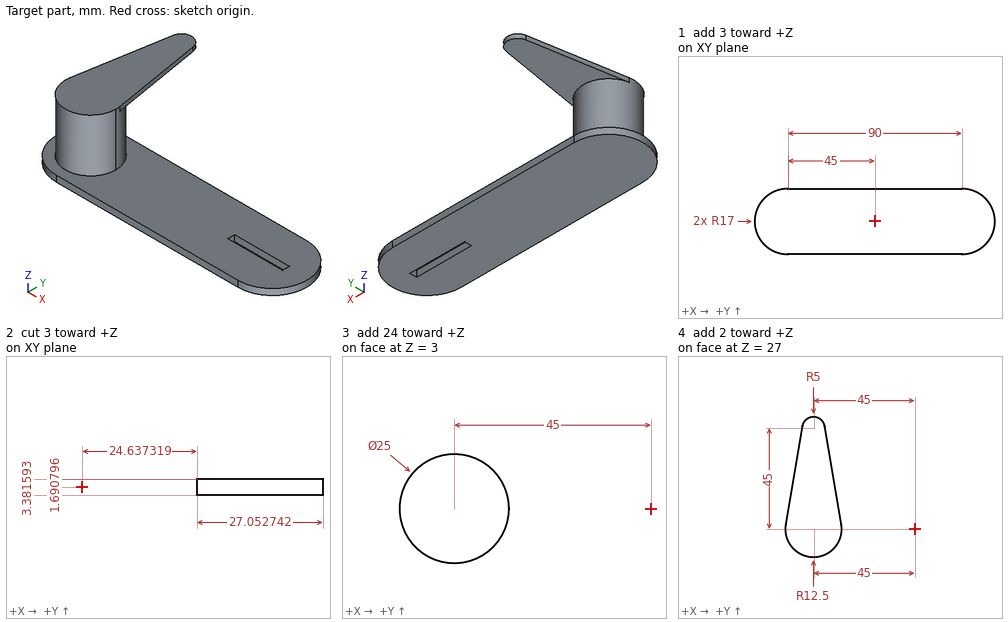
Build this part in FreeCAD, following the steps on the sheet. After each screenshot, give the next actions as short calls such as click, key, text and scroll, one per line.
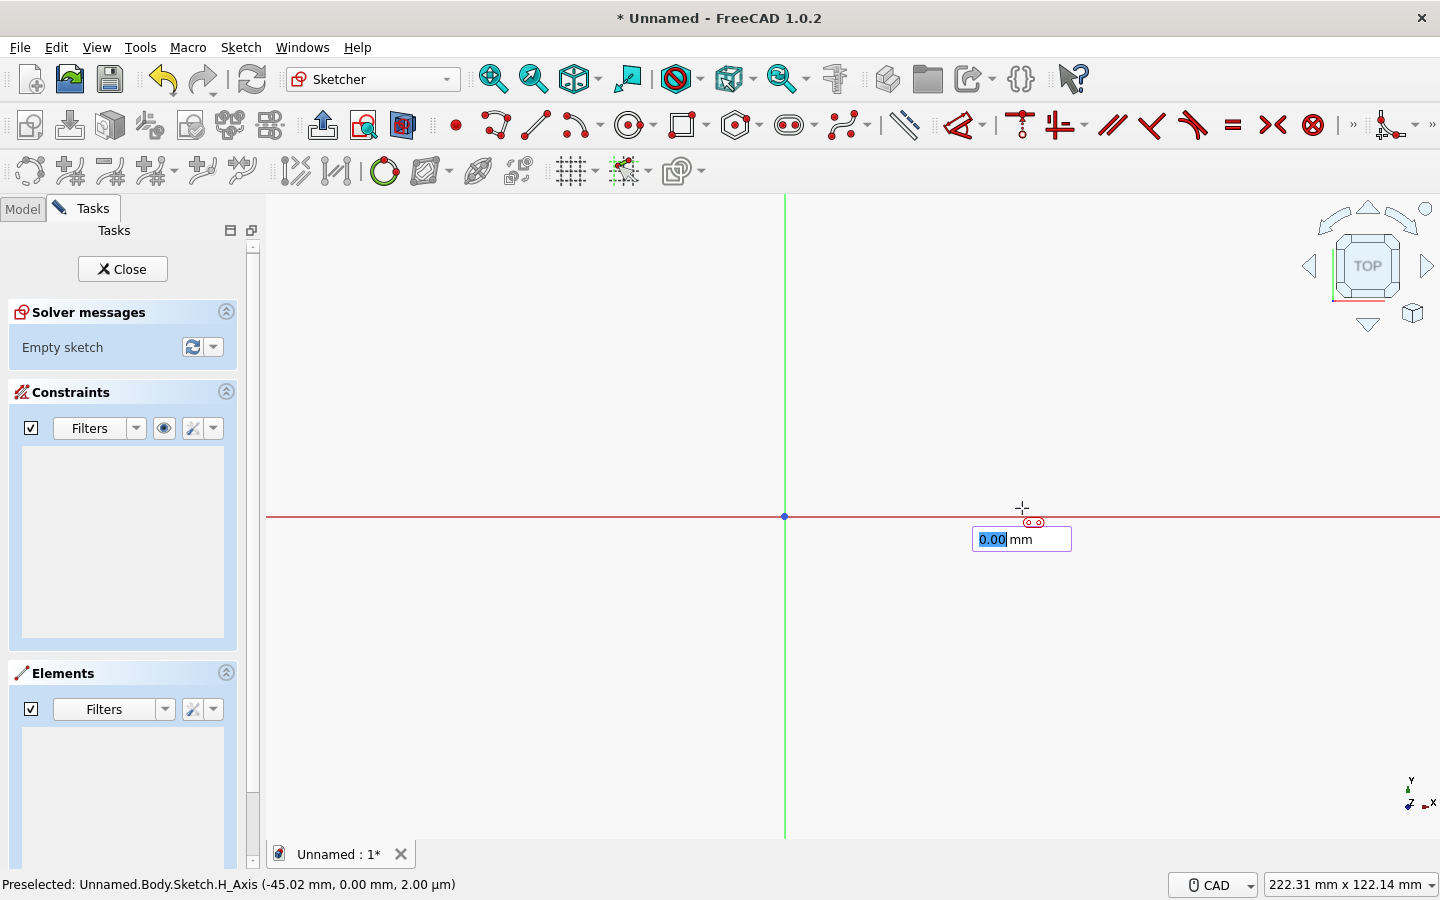
click(856, 427)
key(Escape)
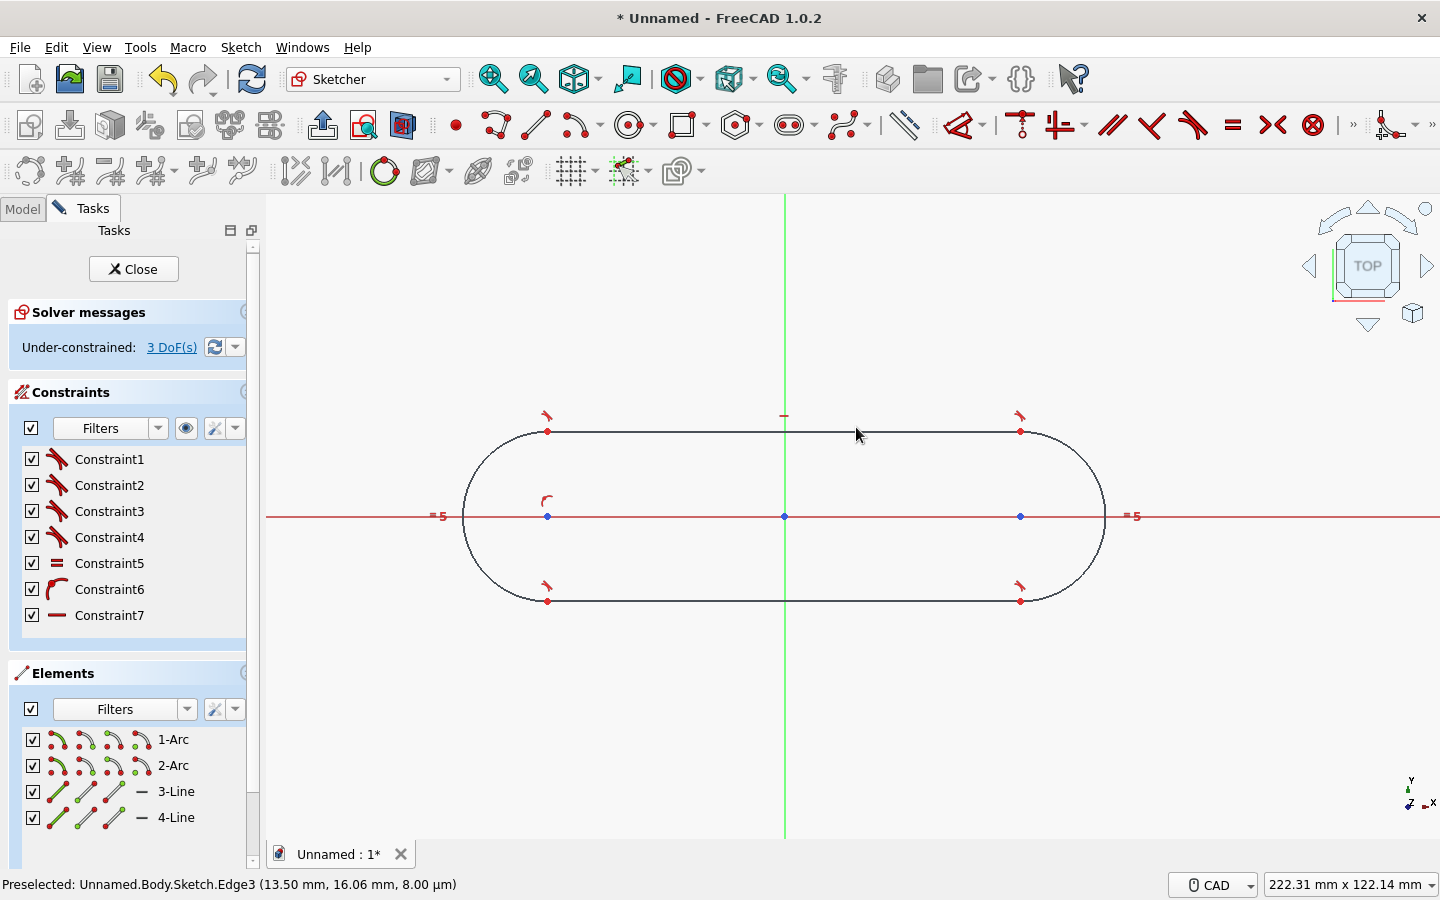
click(958, 126)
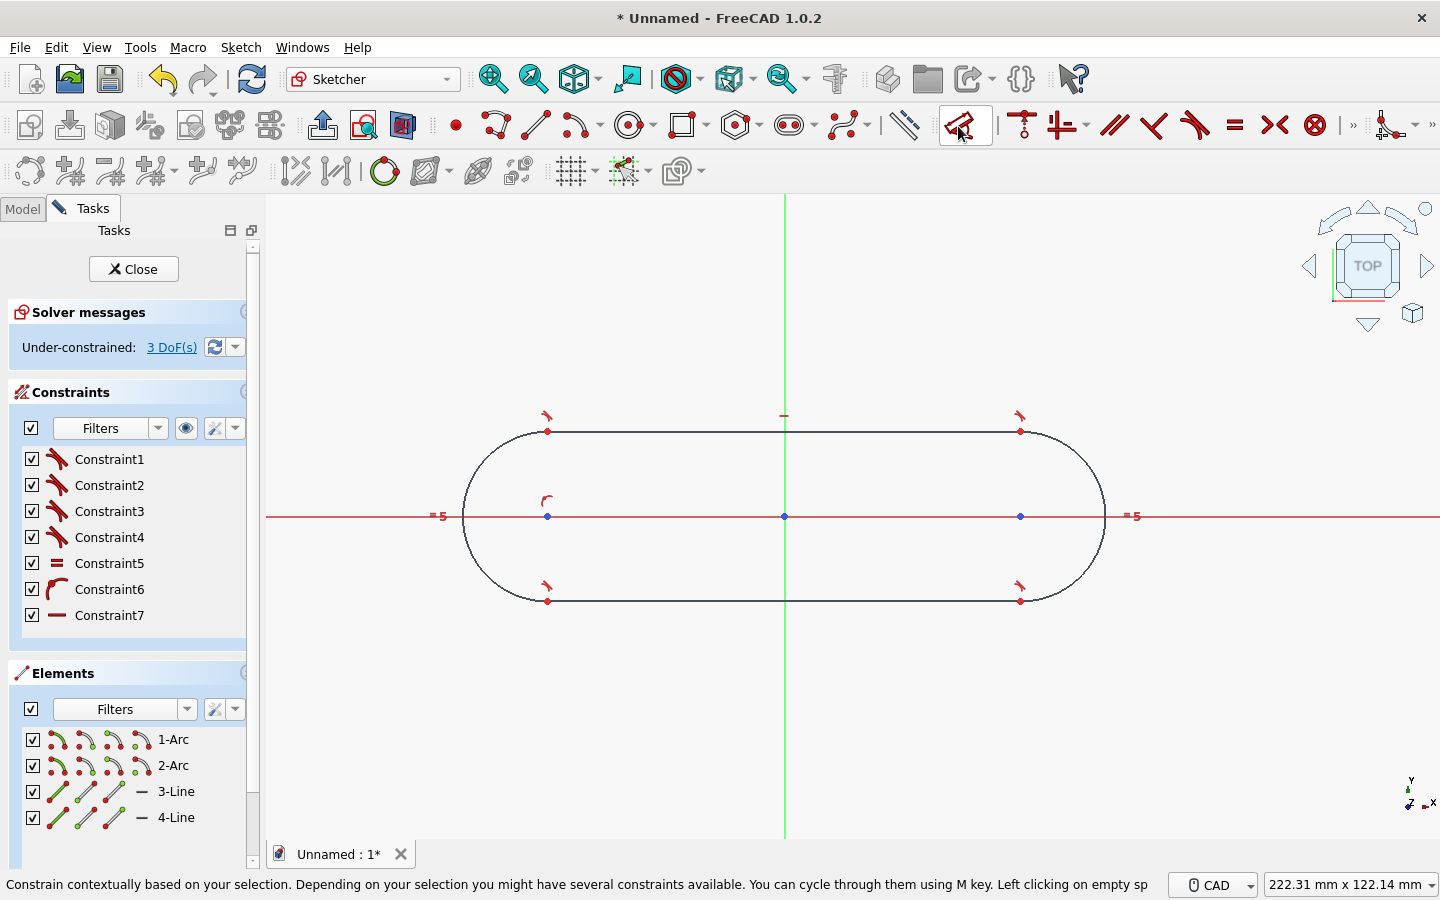
click(479, 467)
click(453, 448)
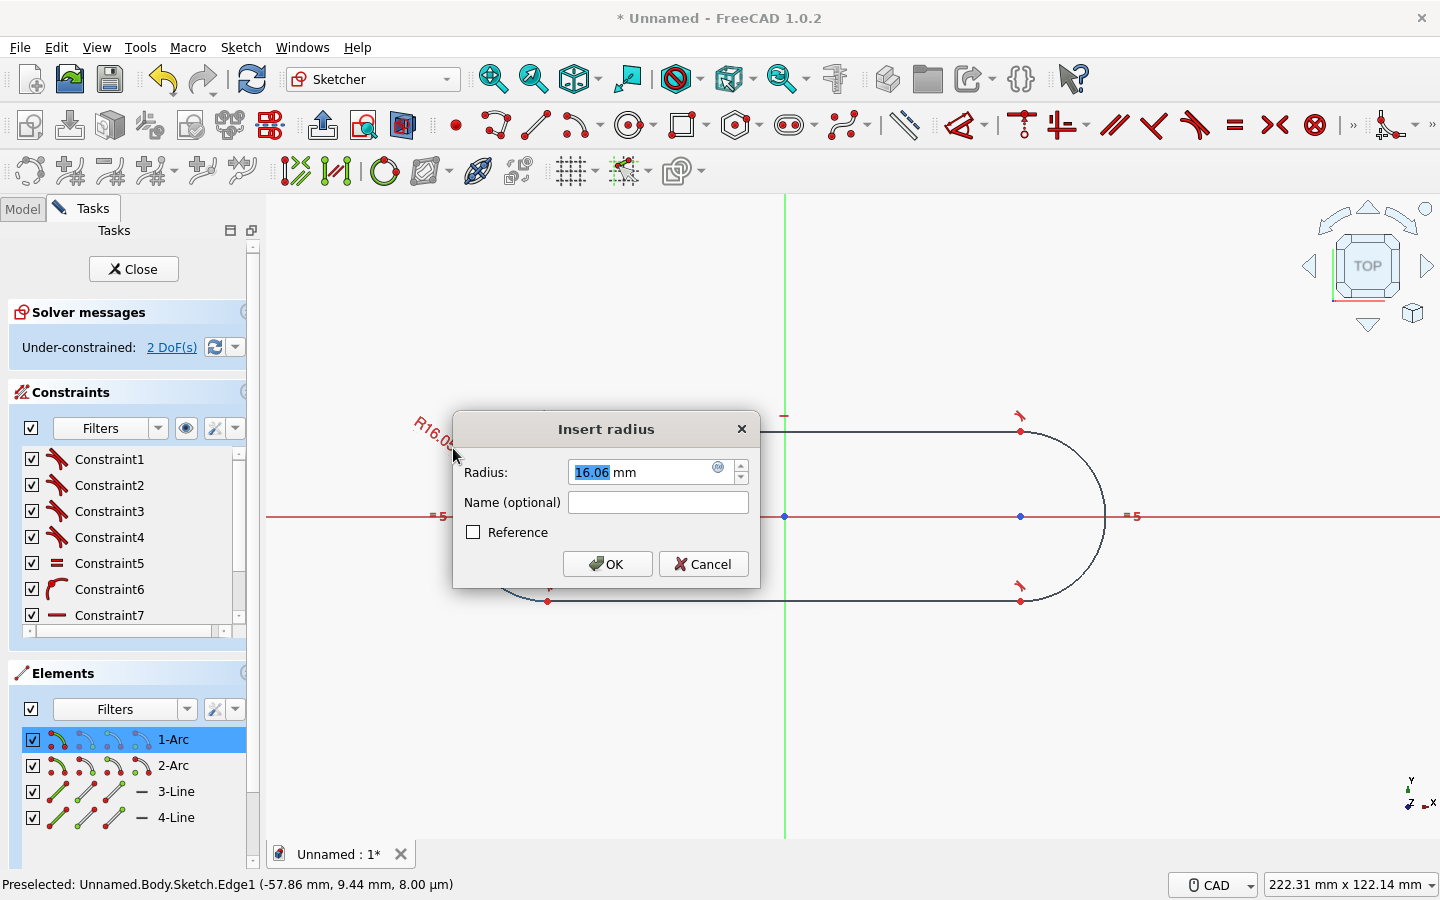
text(17)
key(Return)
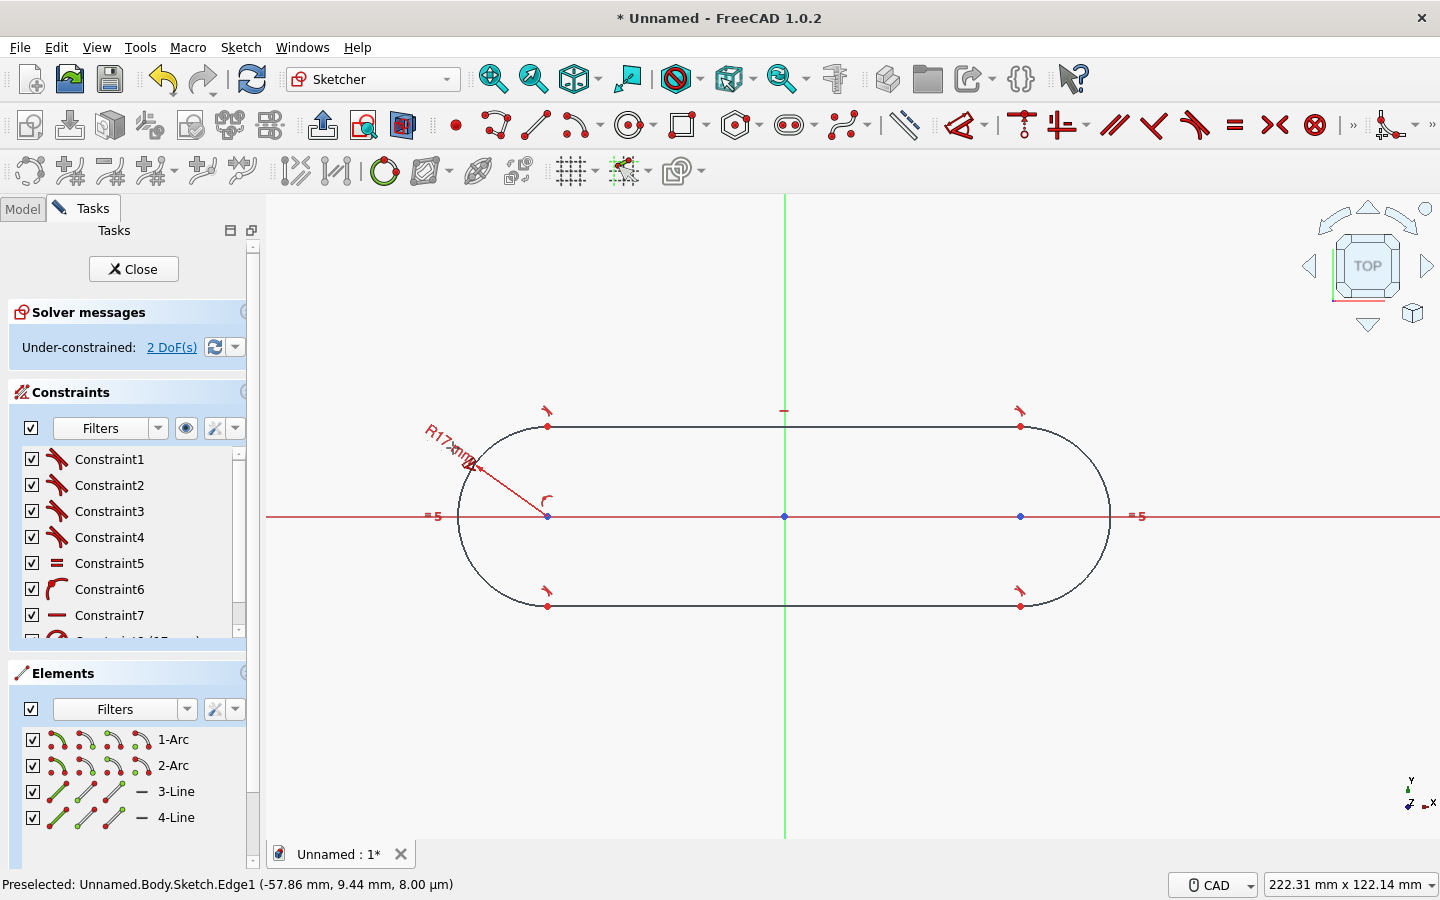
click(690, 427)
click(675, 393)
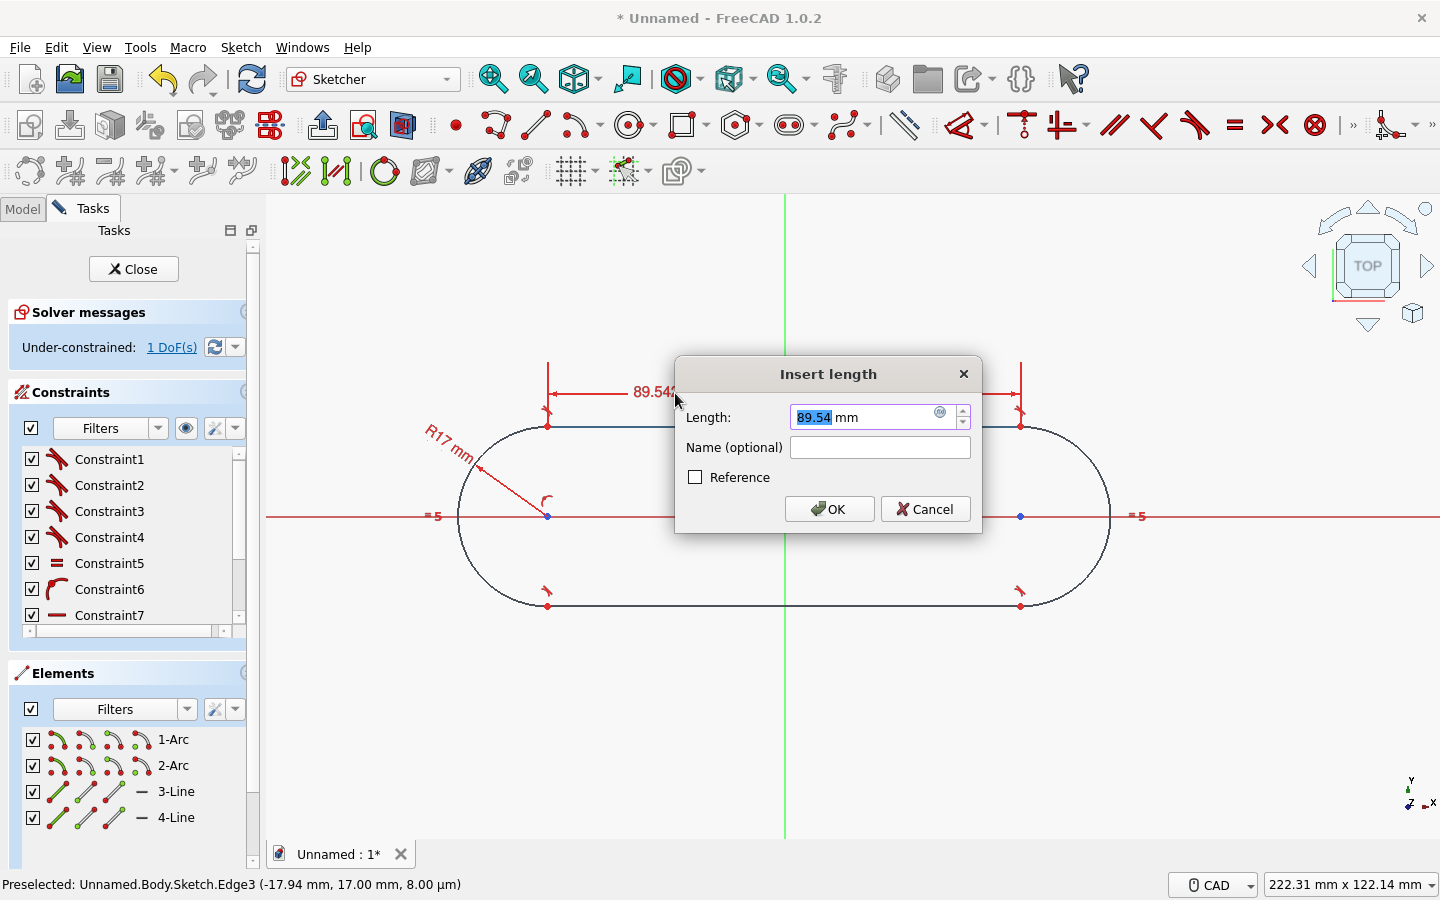
text(90)
key(Return)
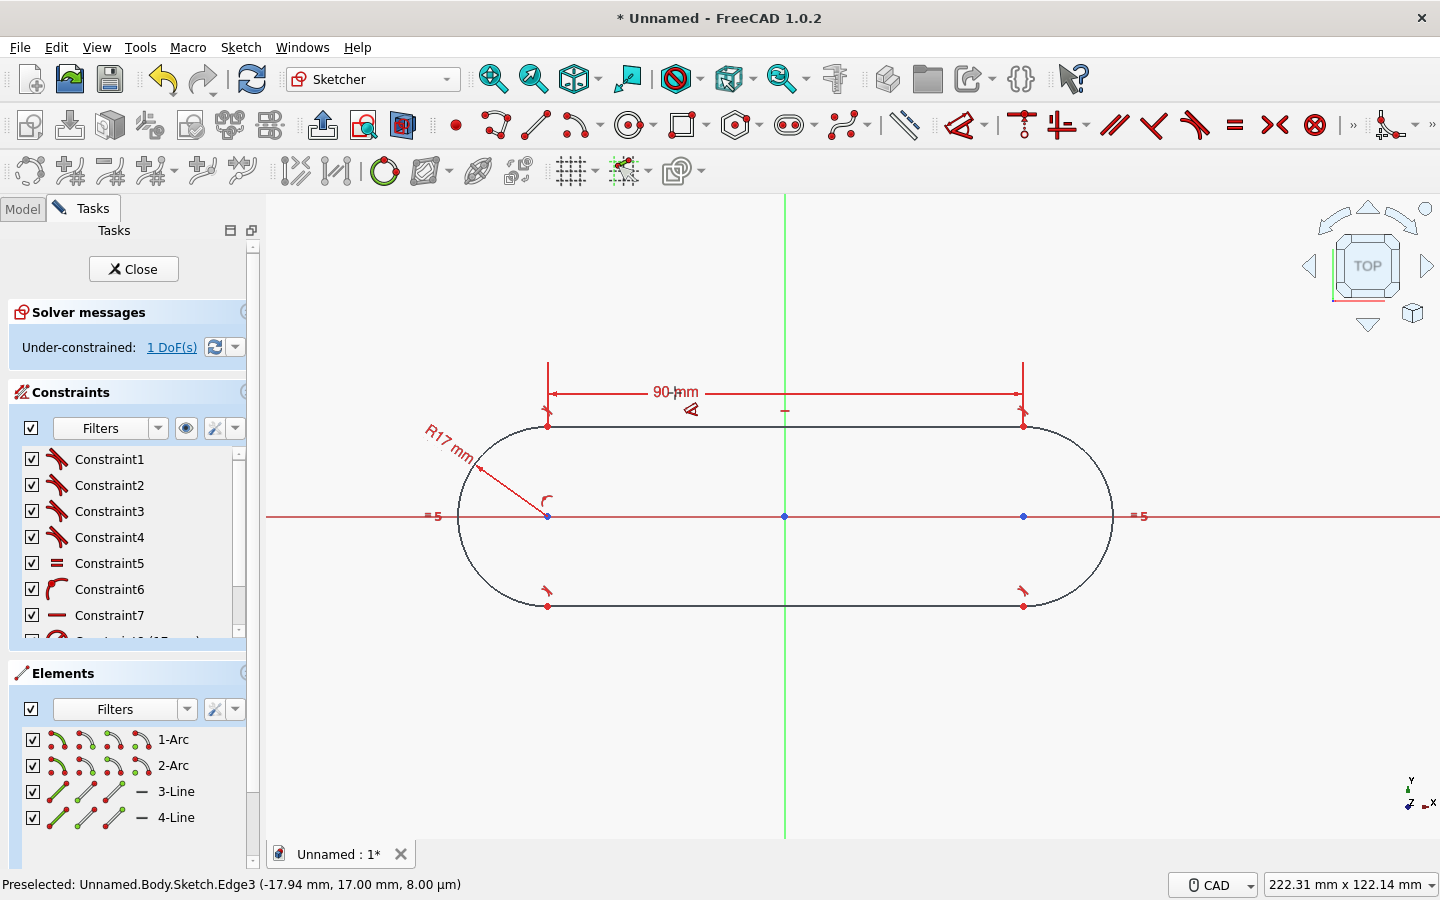
click(548, 427)
click(583, 393)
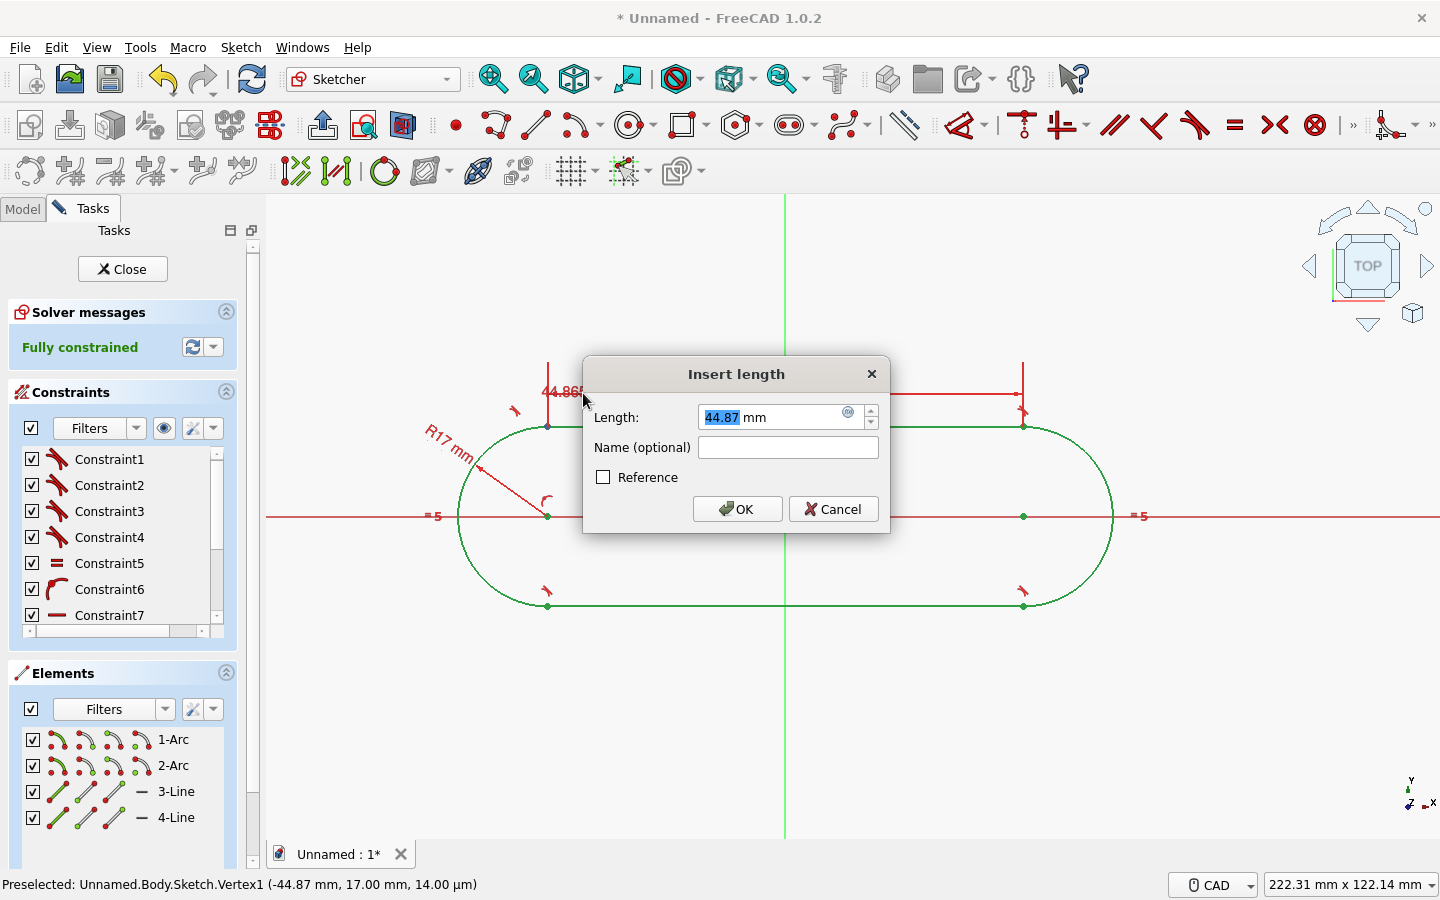
text(45)
key(Return)
key(Escape)